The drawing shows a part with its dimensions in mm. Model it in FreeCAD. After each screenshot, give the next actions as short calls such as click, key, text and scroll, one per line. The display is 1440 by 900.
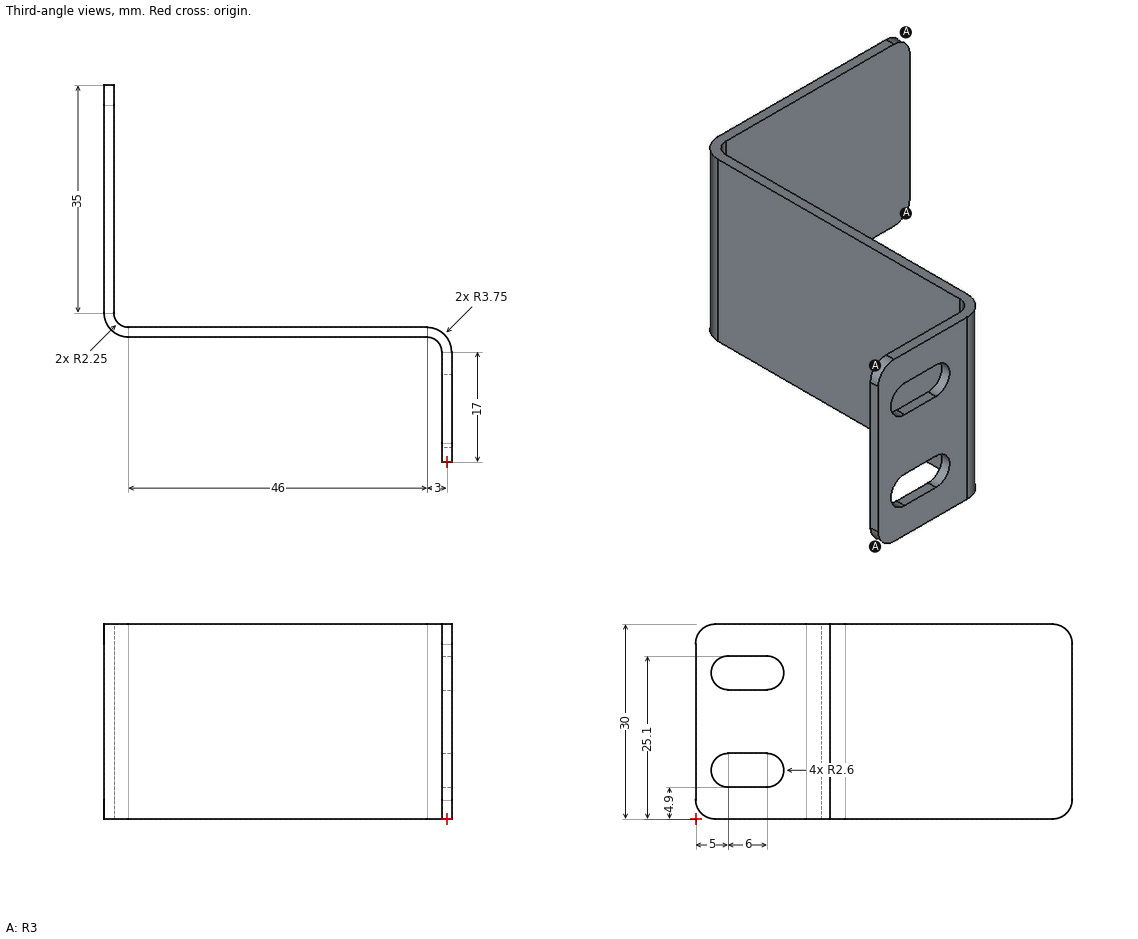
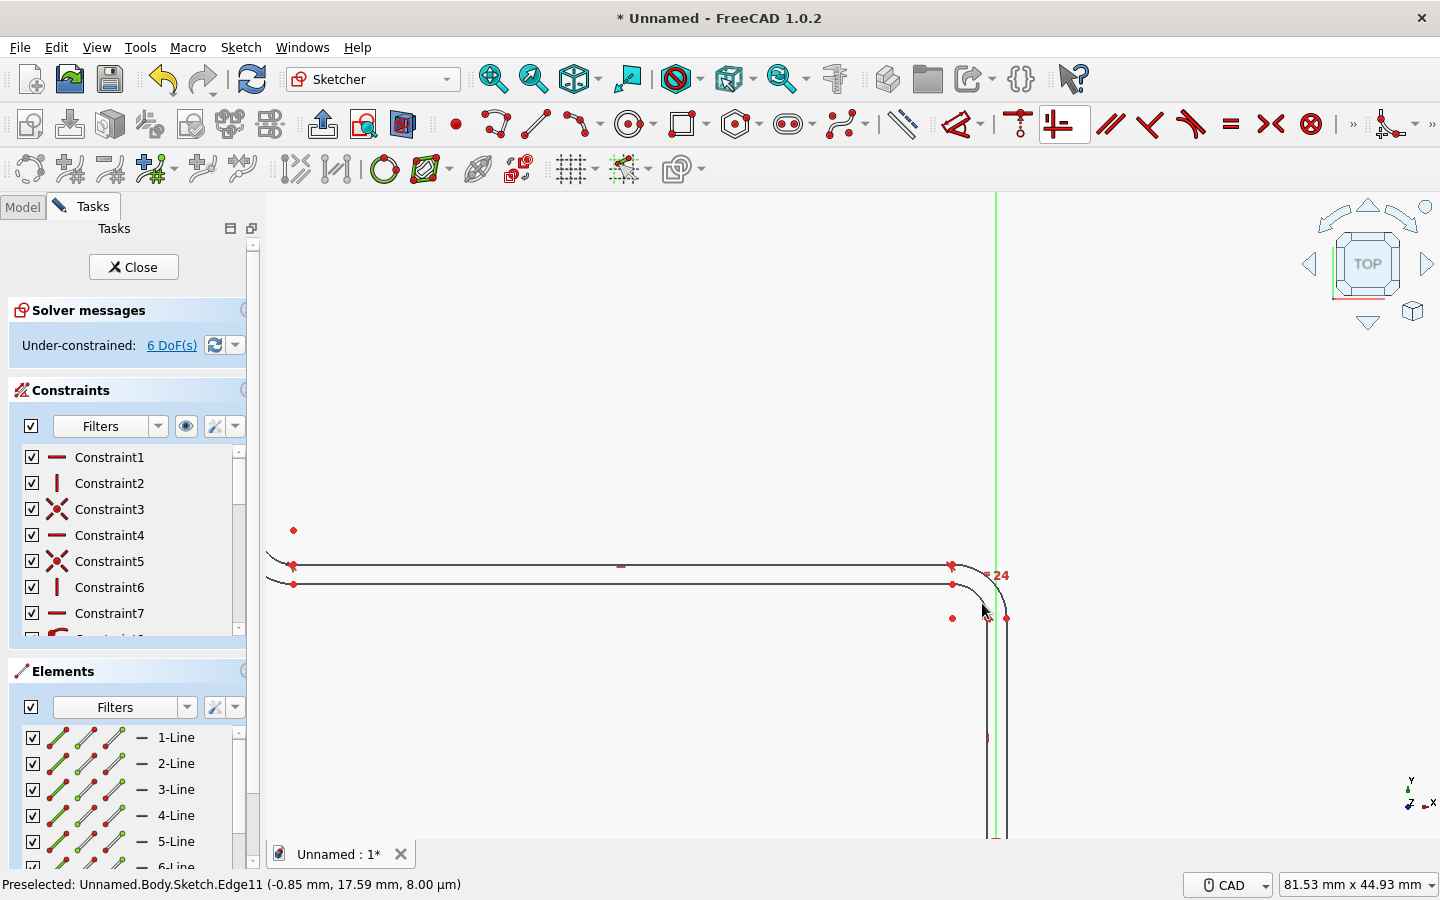
click(956, 124)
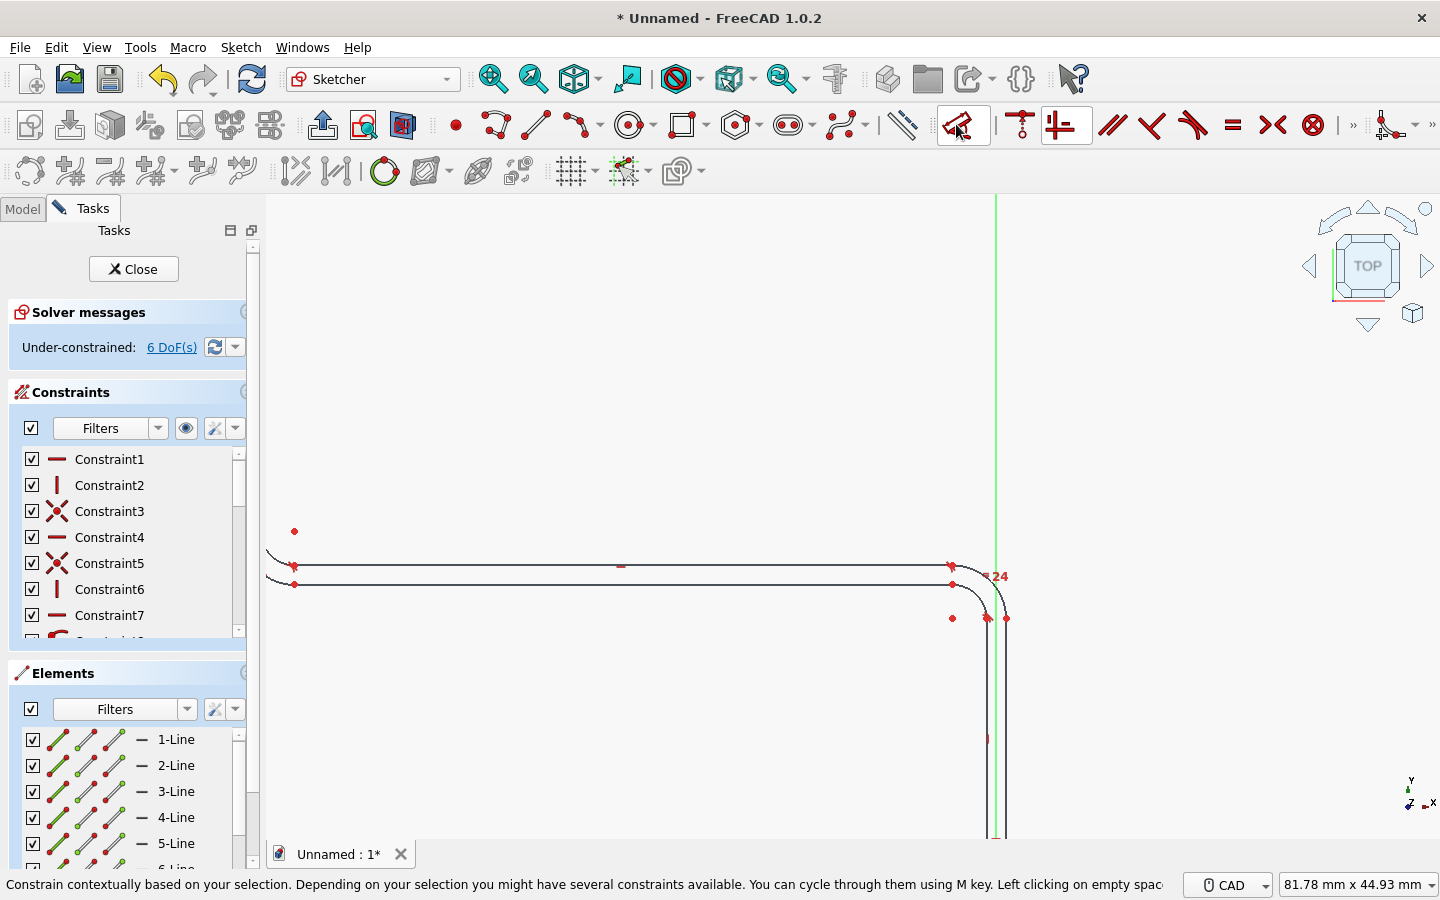
scroll(981, 604, down, 3)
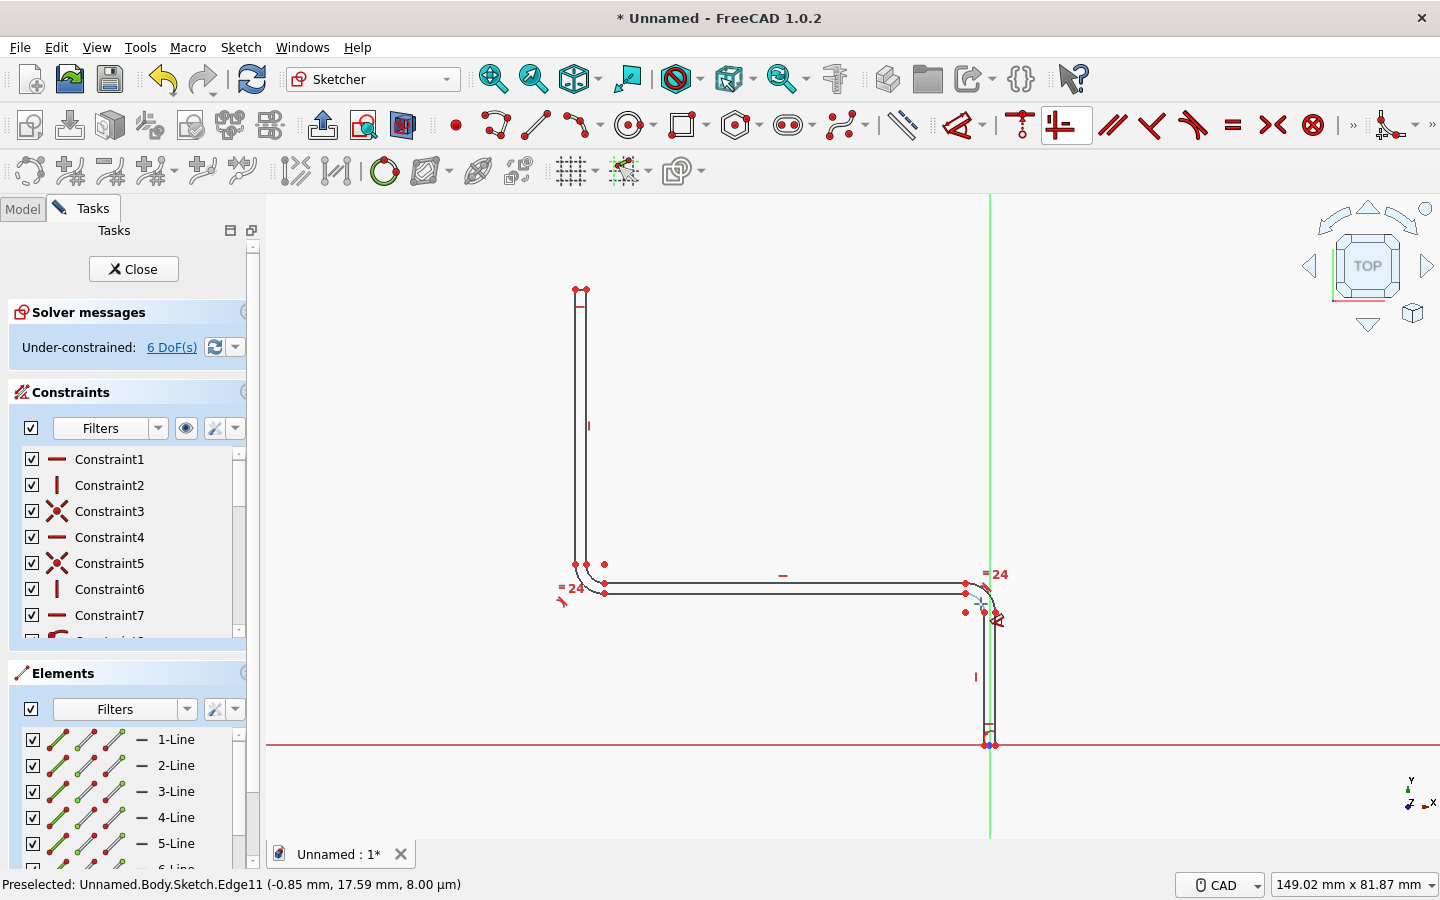
scroll(588, 573, up, 5)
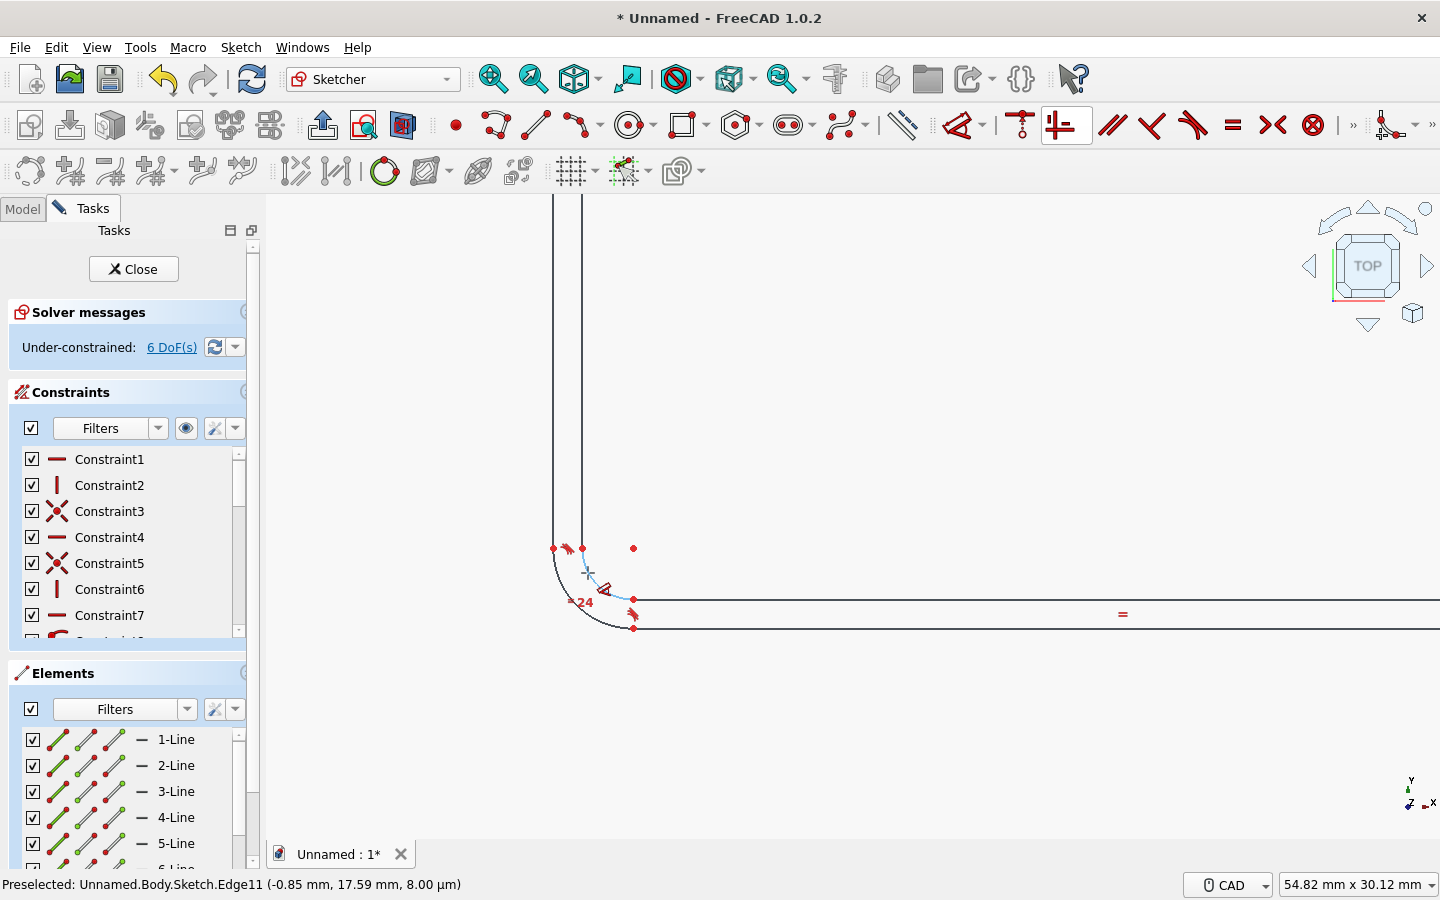
click(588, 572)
click(707, 511)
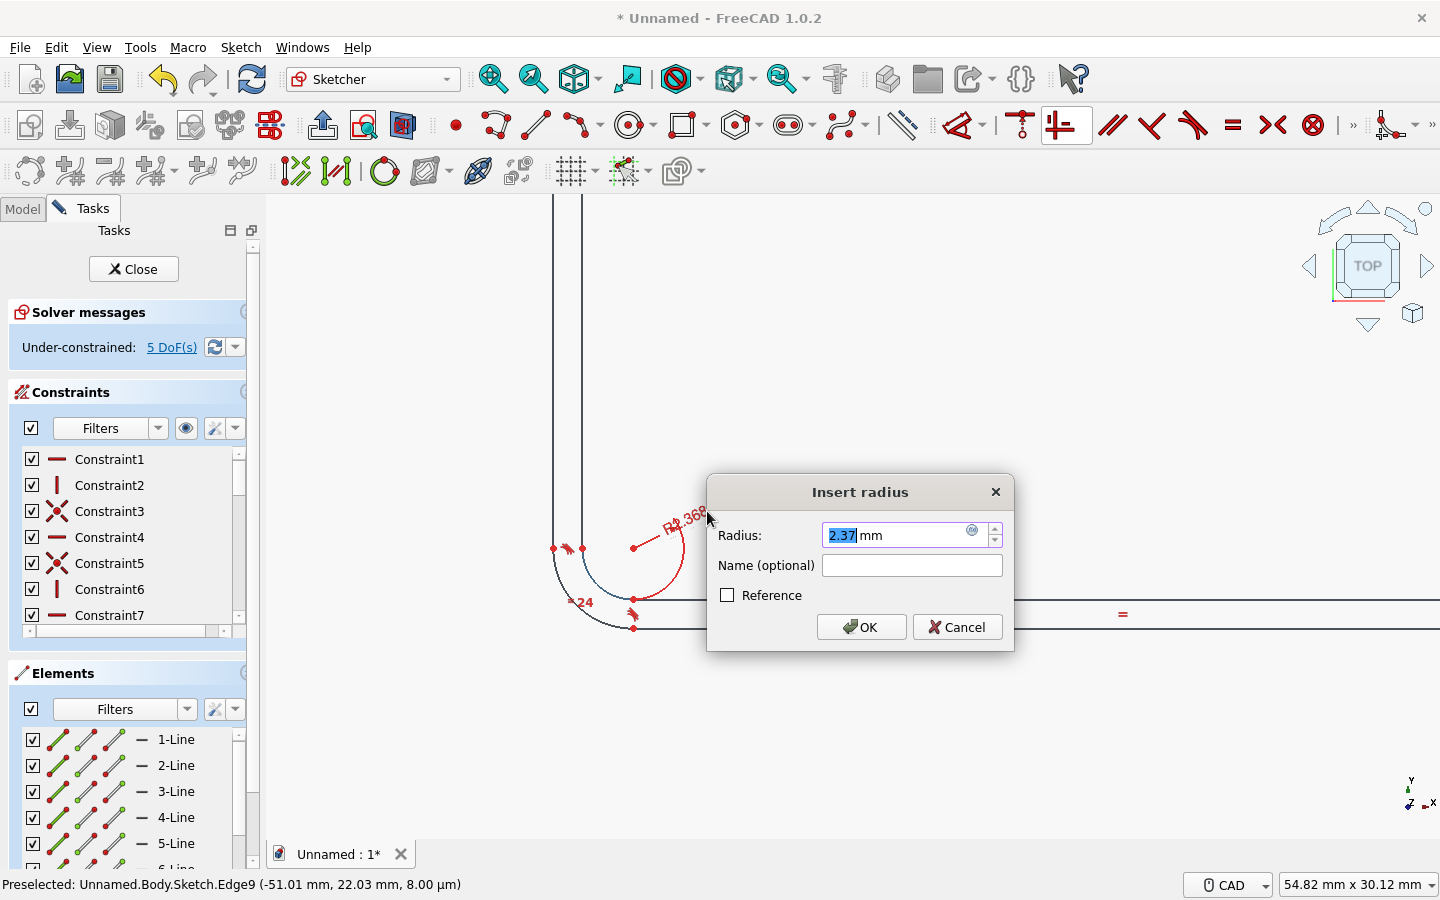
text(2.25)
key(Return)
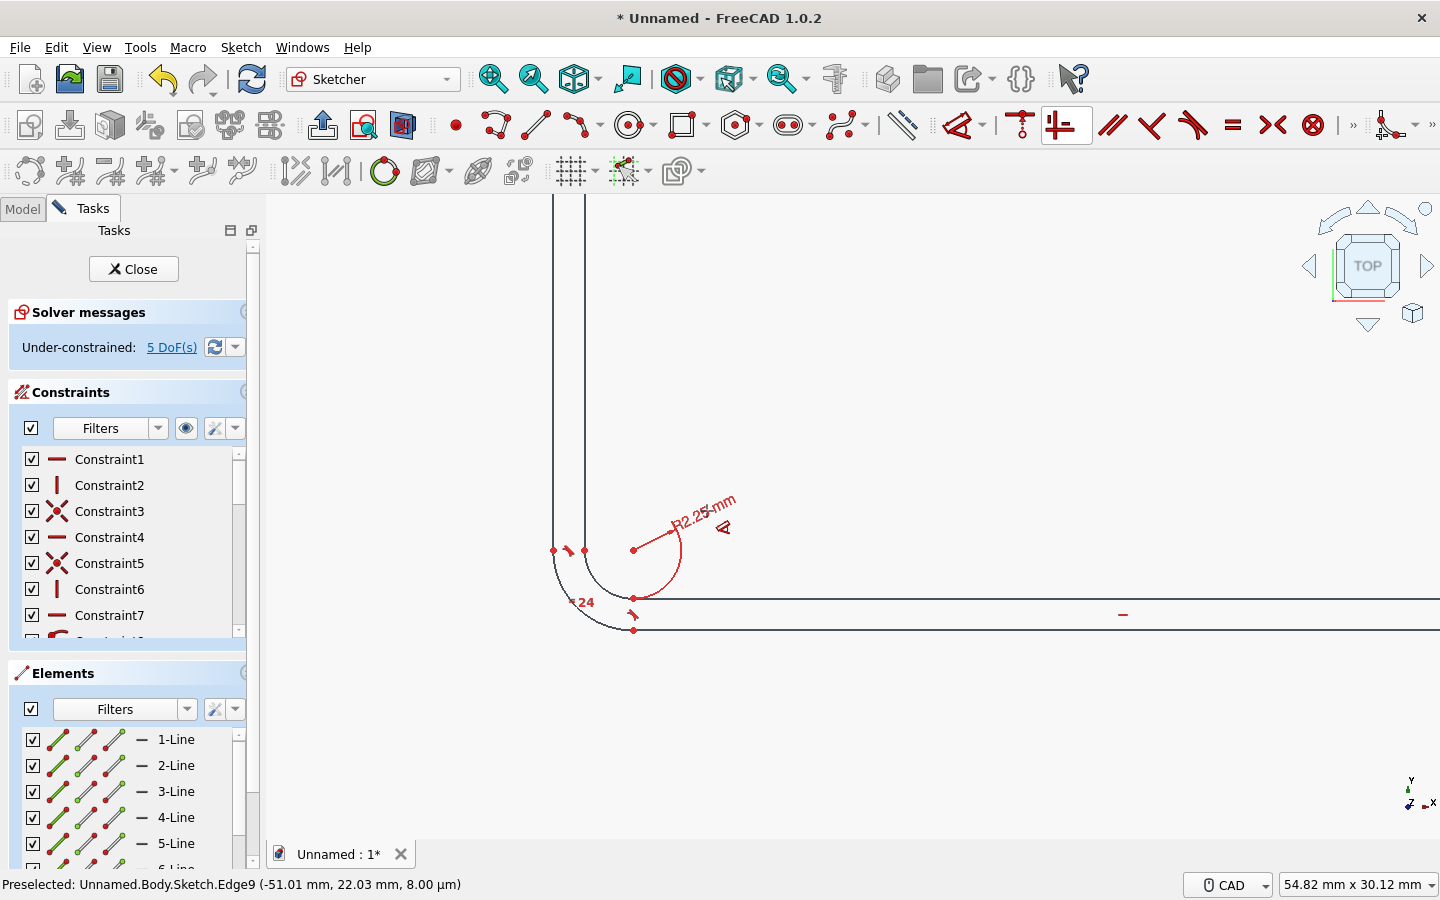
click(562, 587)
click(534, 602)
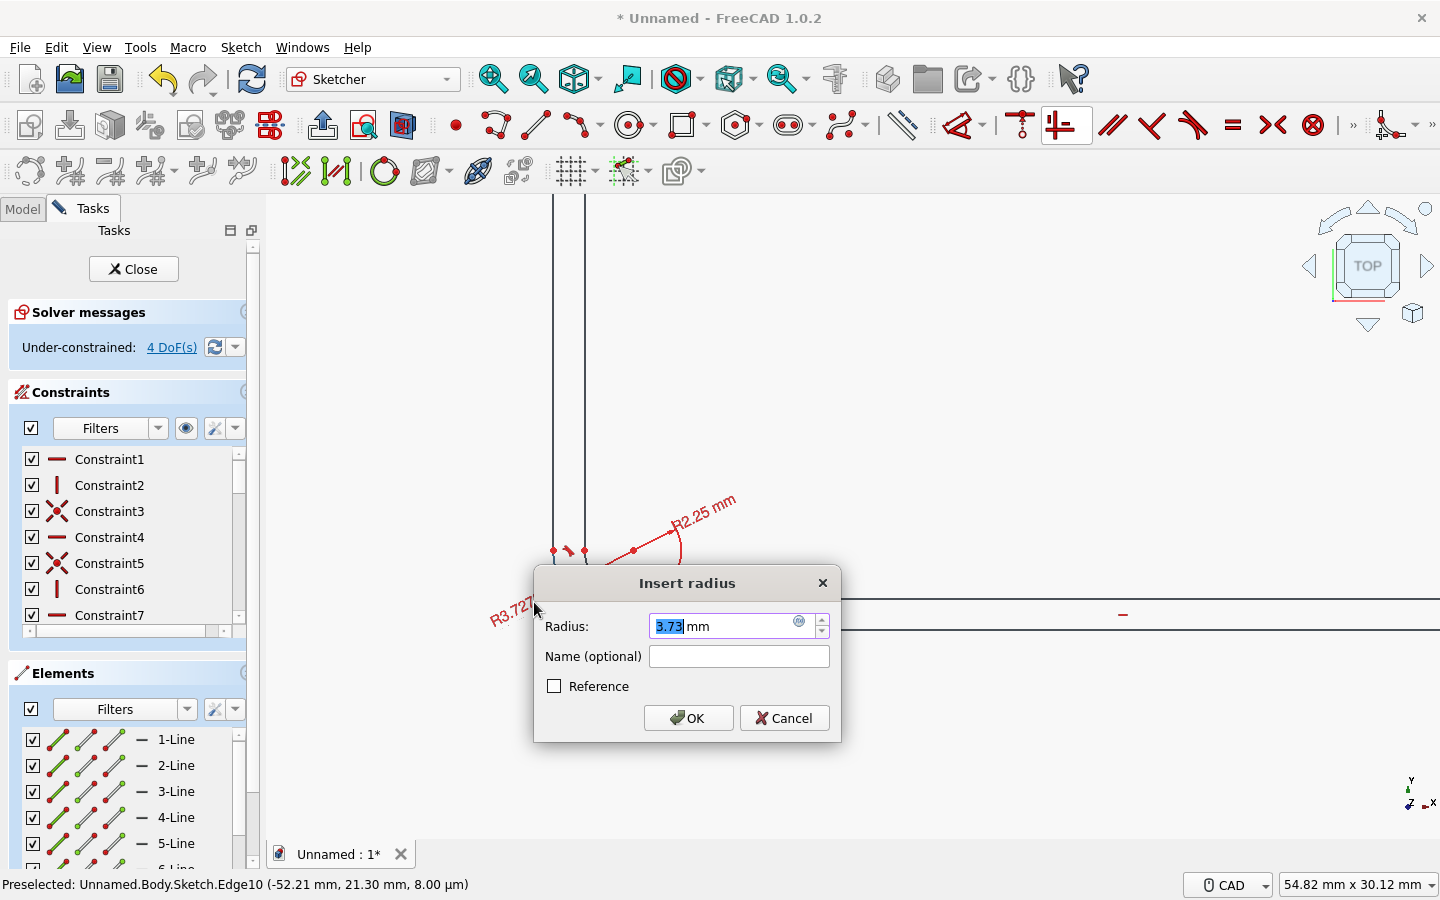
text(3.75)
key(Return)